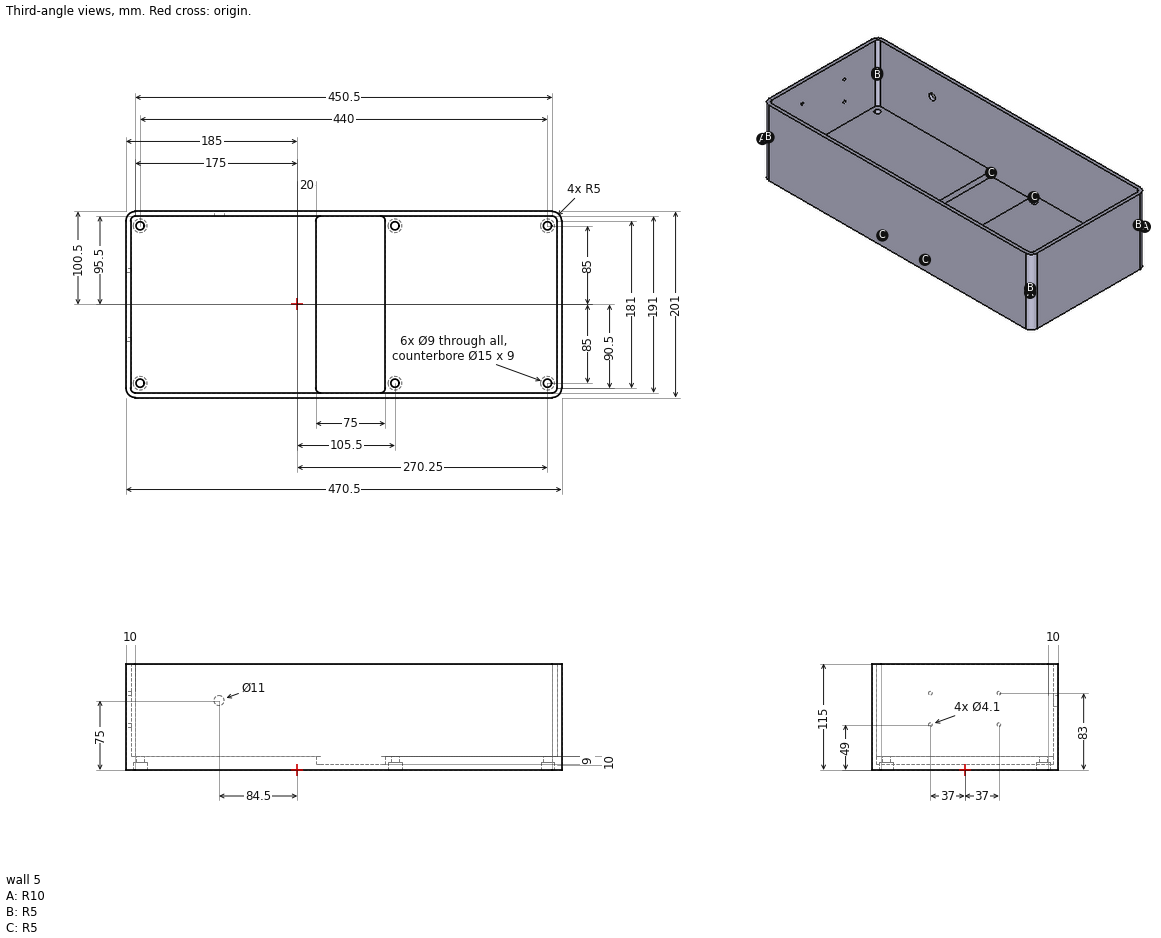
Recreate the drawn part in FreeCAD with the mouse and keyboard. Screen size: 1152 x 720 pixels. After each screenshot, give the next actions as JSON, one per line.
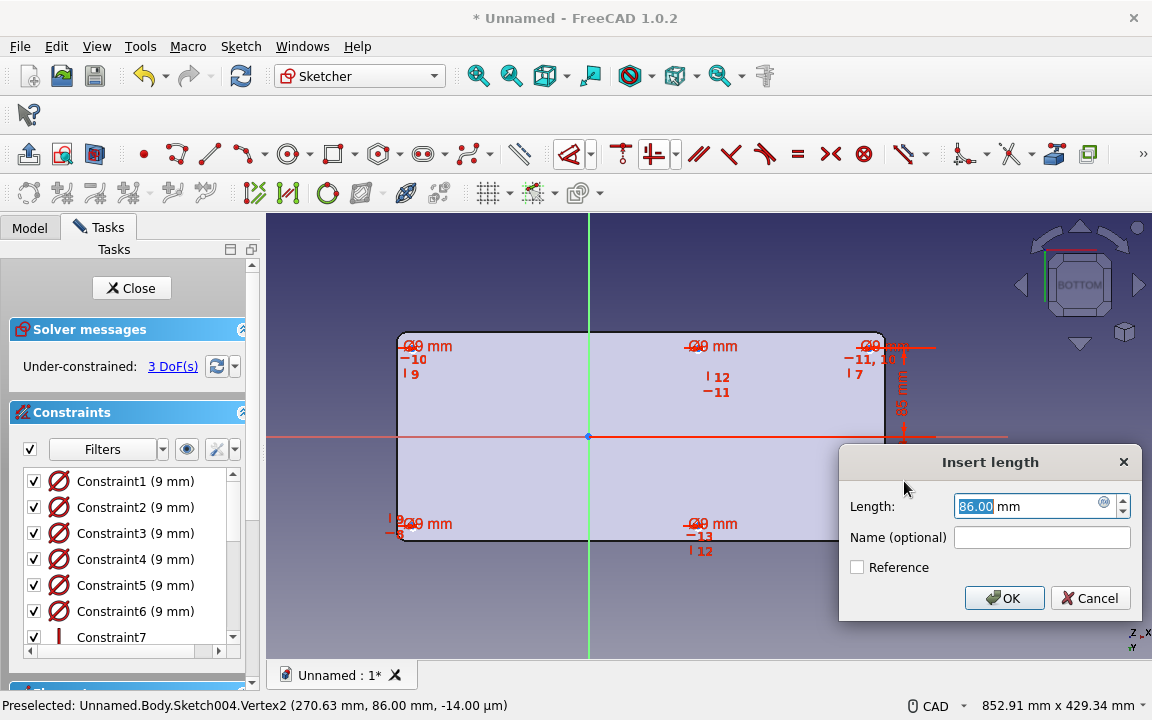
{"action": "type", "text": "85"}
{"action": "key", "text": "Return"}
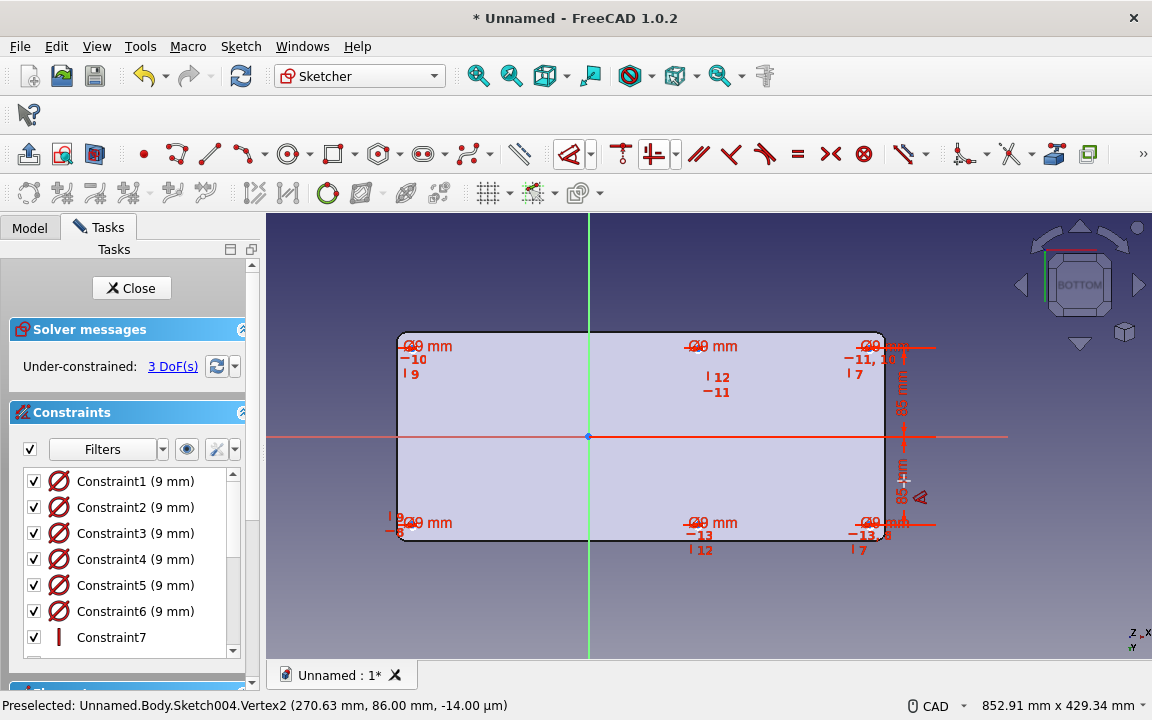
{"action": "left_click", "coordinate": [870, 525]}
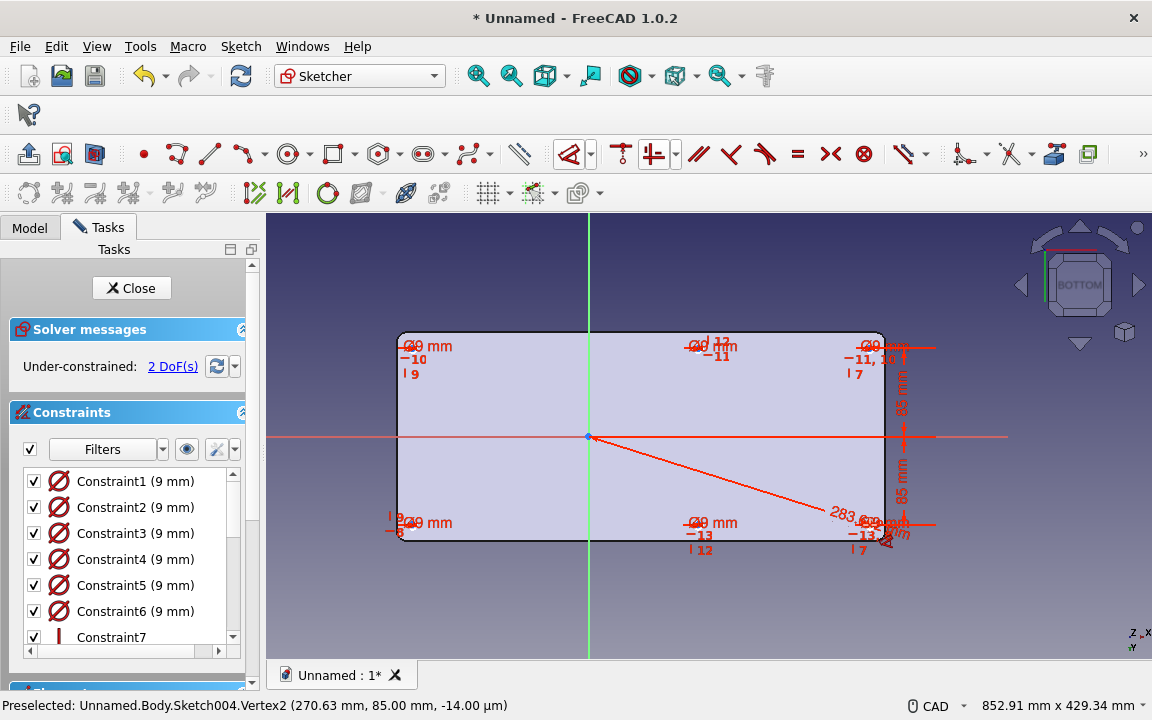
{"action": "left_click", "coordinate": [413, 525]}
{"action": "left_click", "coordinate": [641, 559]}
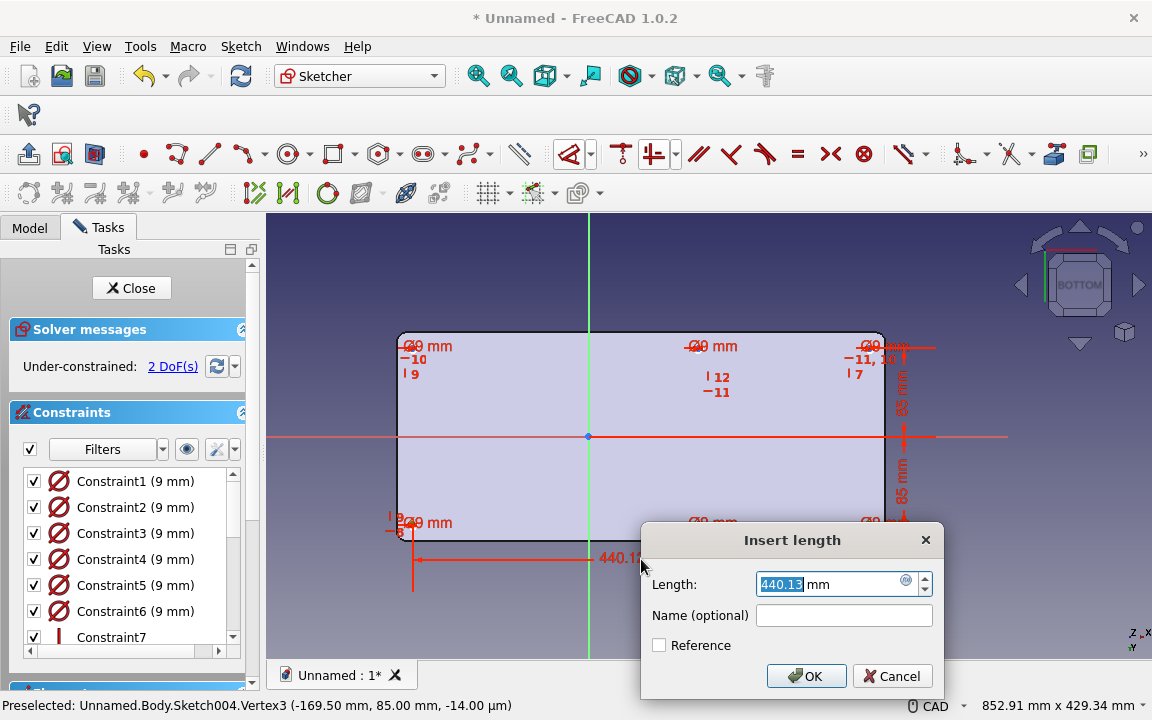
{"action": "type", "text": "440"}
{"action": "key", "text": "Return"}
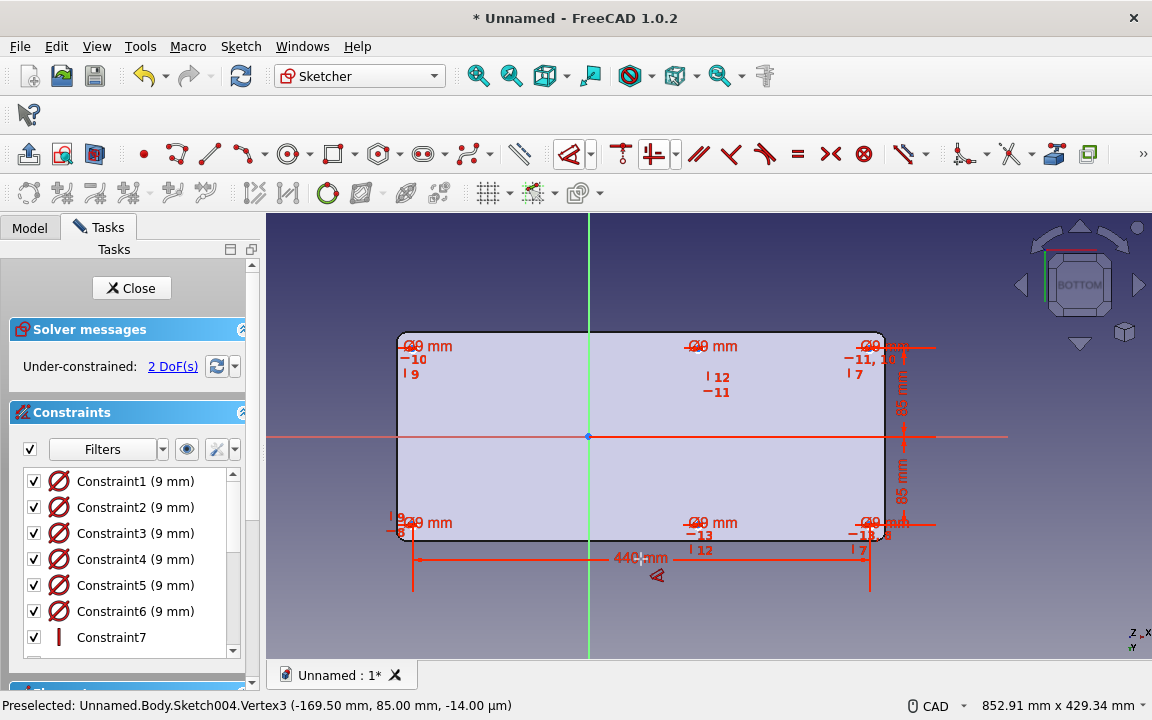
{"action": "left_click", "coordinate": [698, 348]}
{"action": "left_click", "coordinate": [643, 314]}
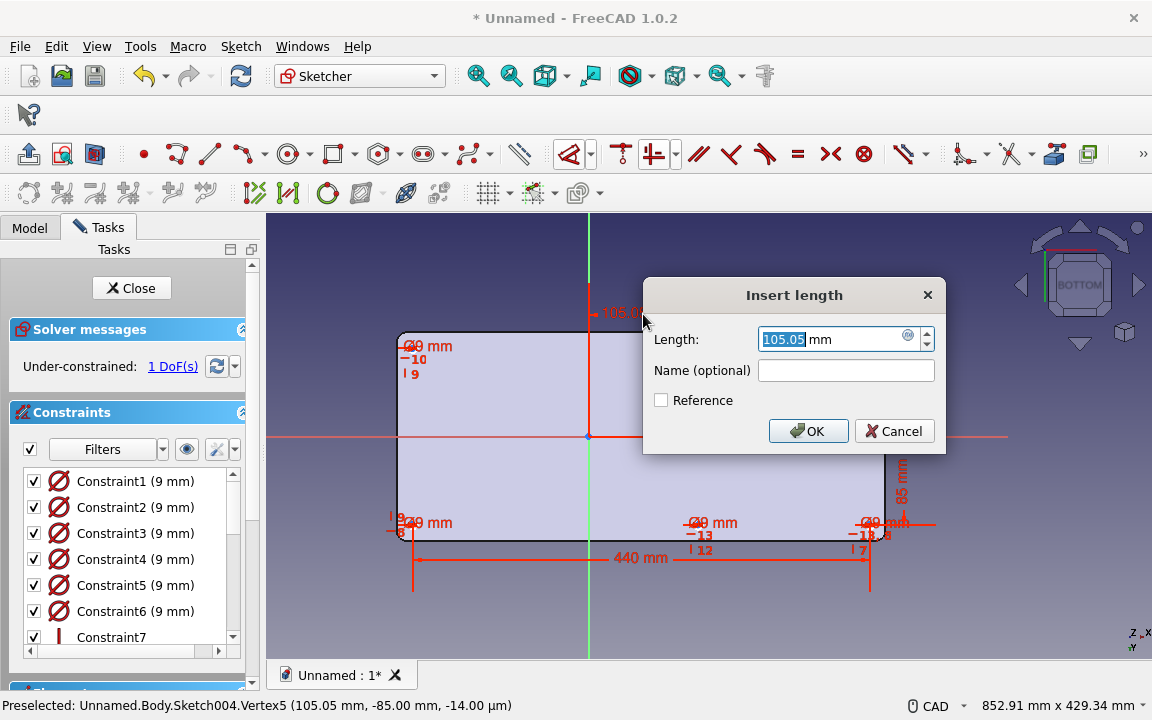
{"action": "type", "text": "105.5"}
{"action": "key", "text": "Return"}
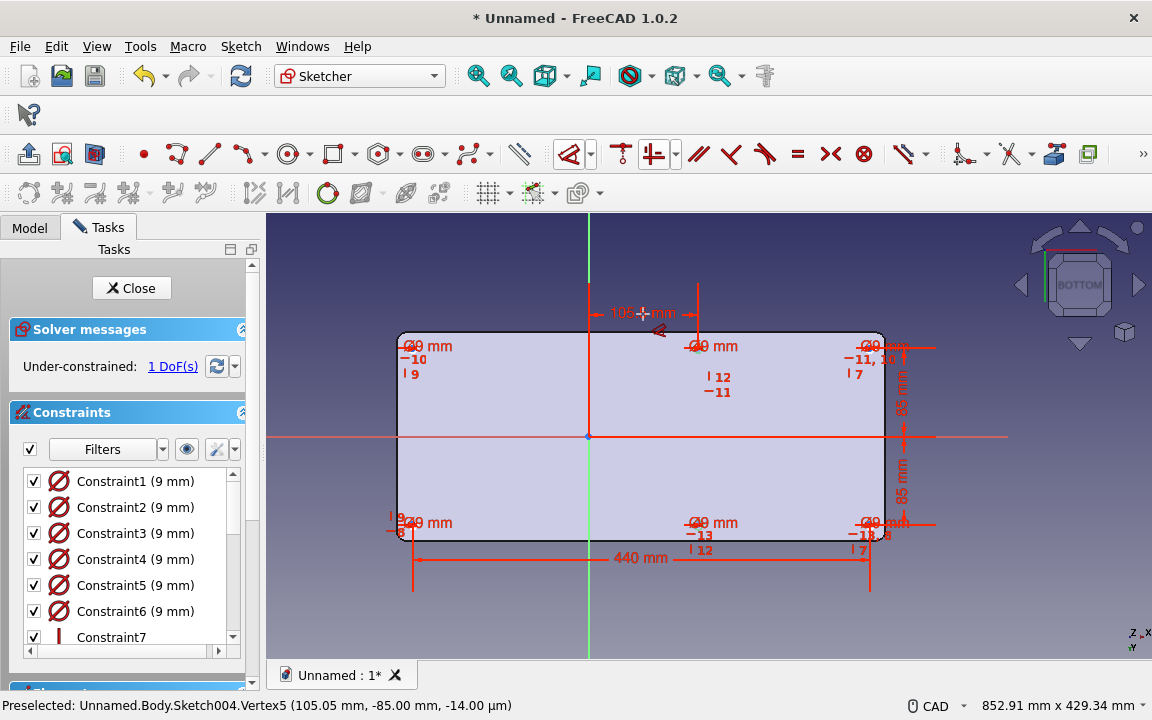
{"action": "left_click", "coordinate": [870, 348]}
{"action": "left_click", "coordinate": [729, 314]}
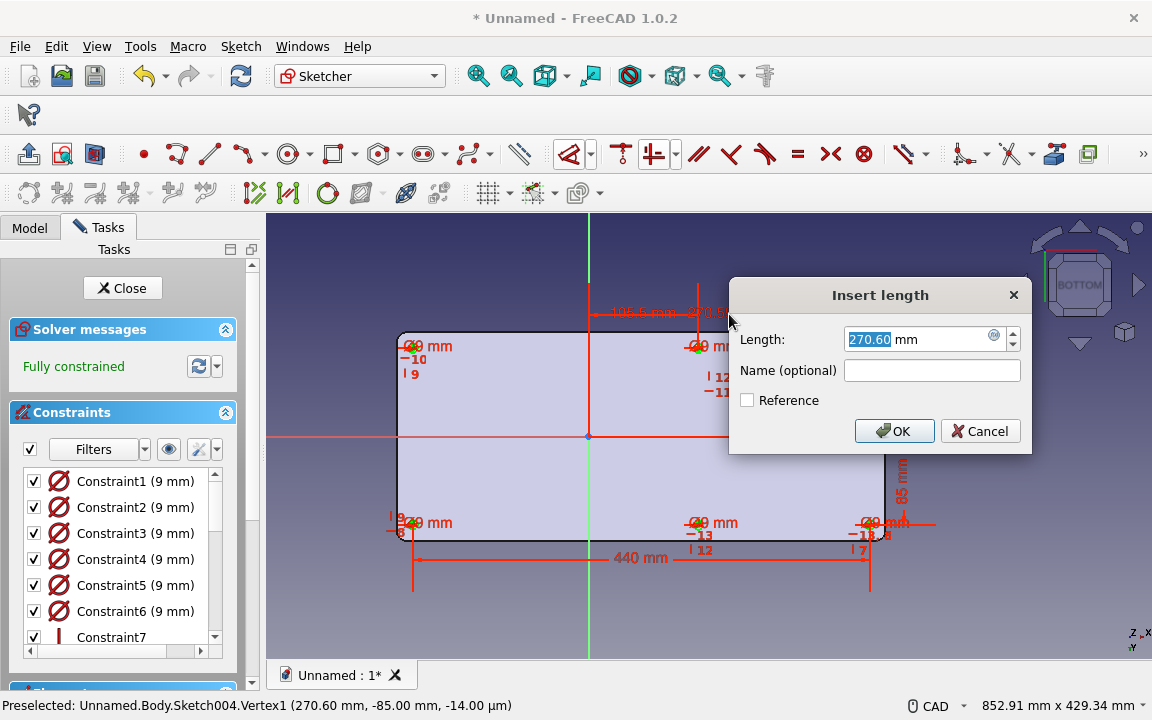
{"action": "type", "text": "270.25"}
{"action": "key", "text": "Return"}
{"action": "key", "text": "Escape"}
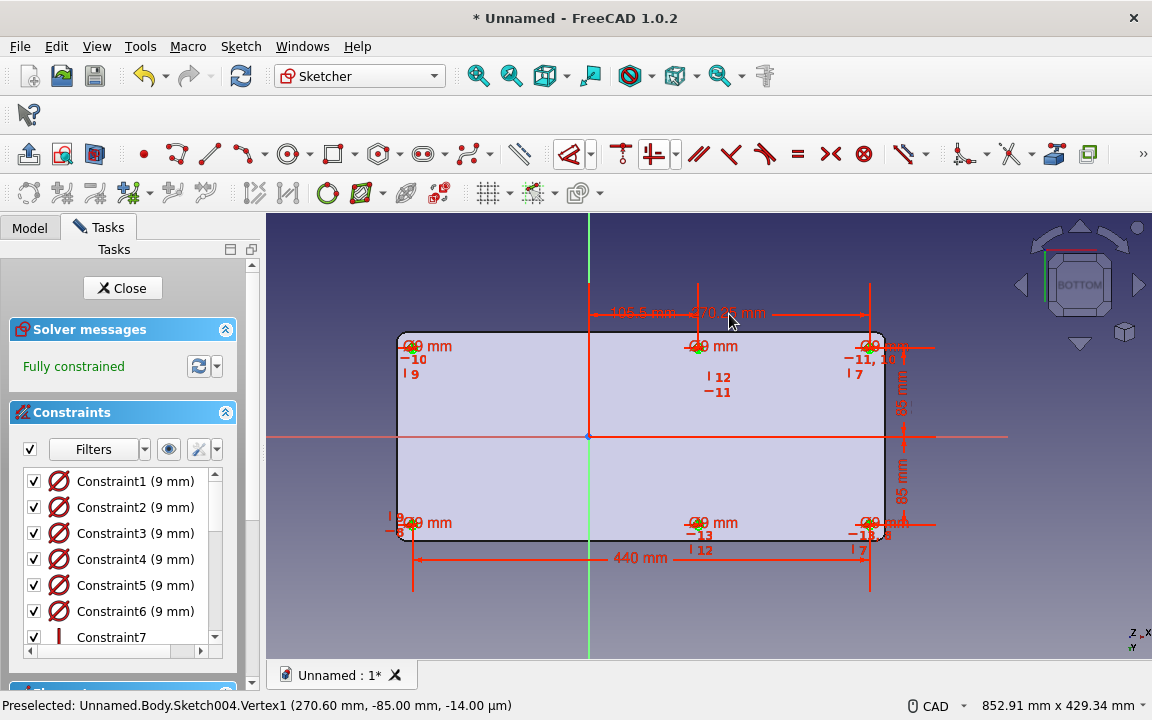
{"action": "left_click", "coordinate": [123, 288]}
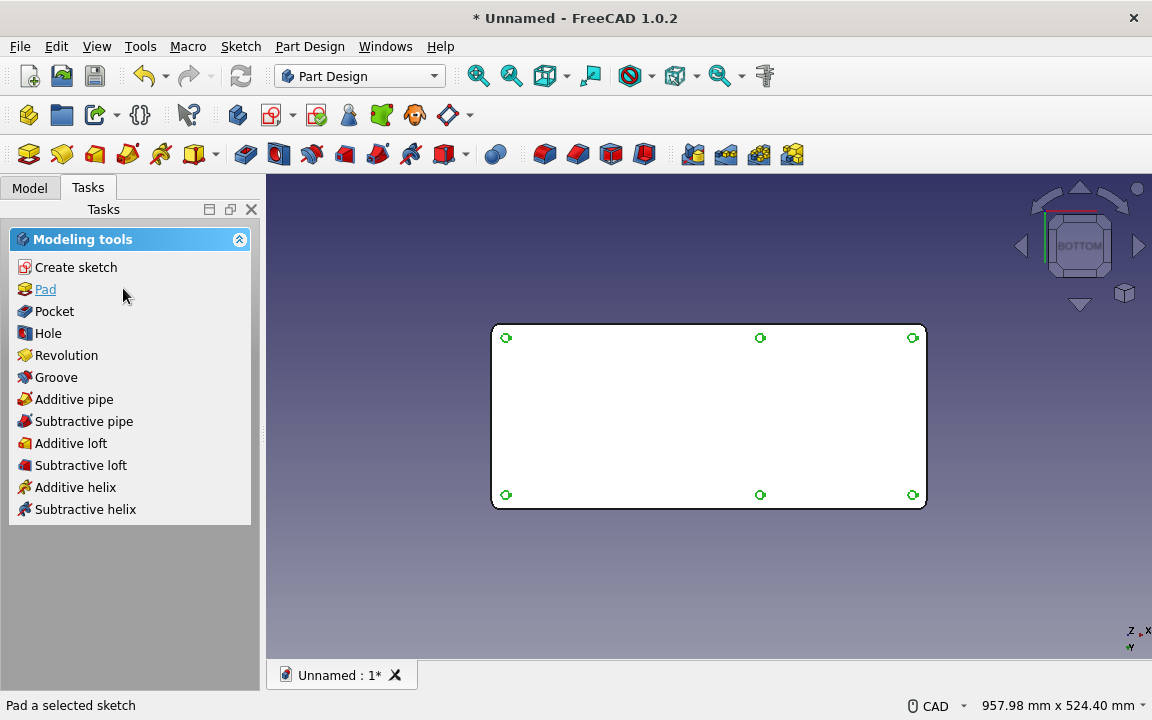
{"action": "left_click", "coordinate": [279, 154]}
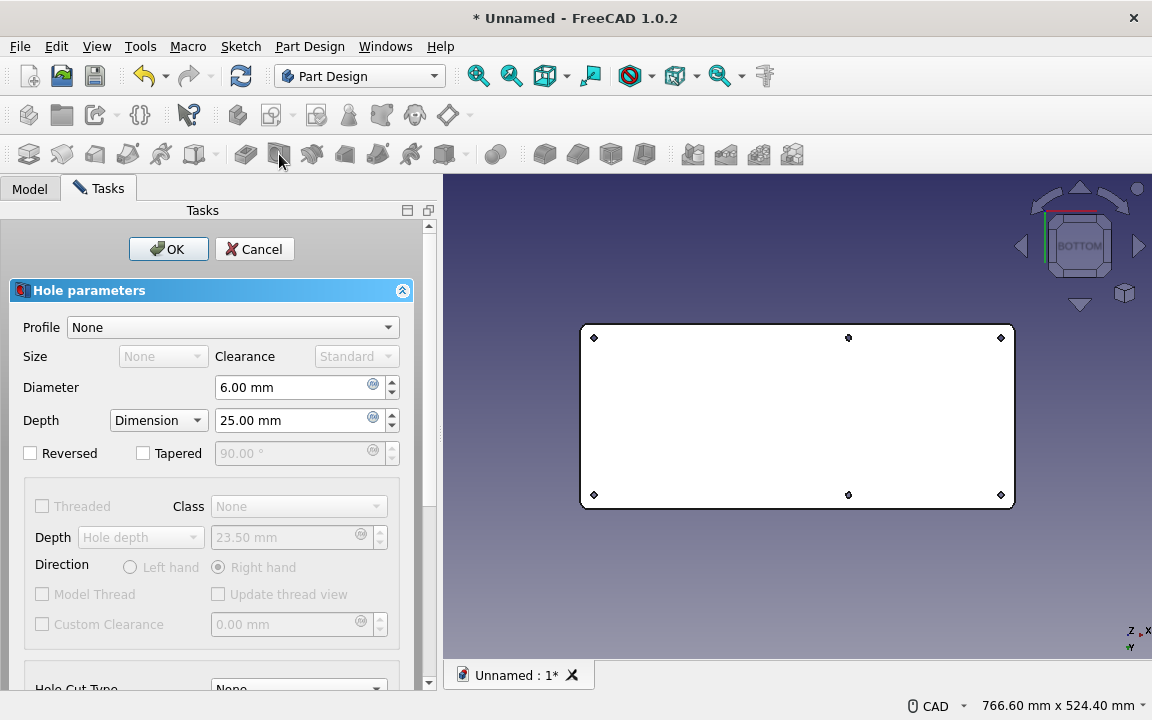
{"action": "triple_click", "coordinate": [300, 388]}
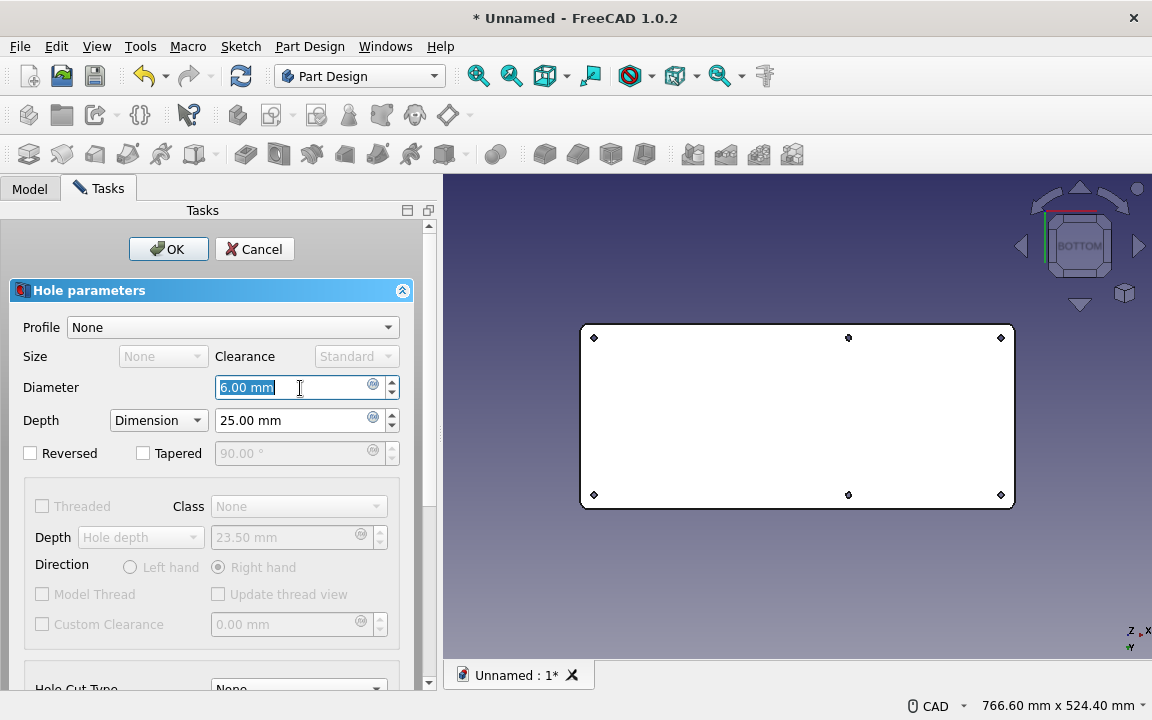
{"action": "type", "text": "9"}
{"action": "key", "text": "Tab"}